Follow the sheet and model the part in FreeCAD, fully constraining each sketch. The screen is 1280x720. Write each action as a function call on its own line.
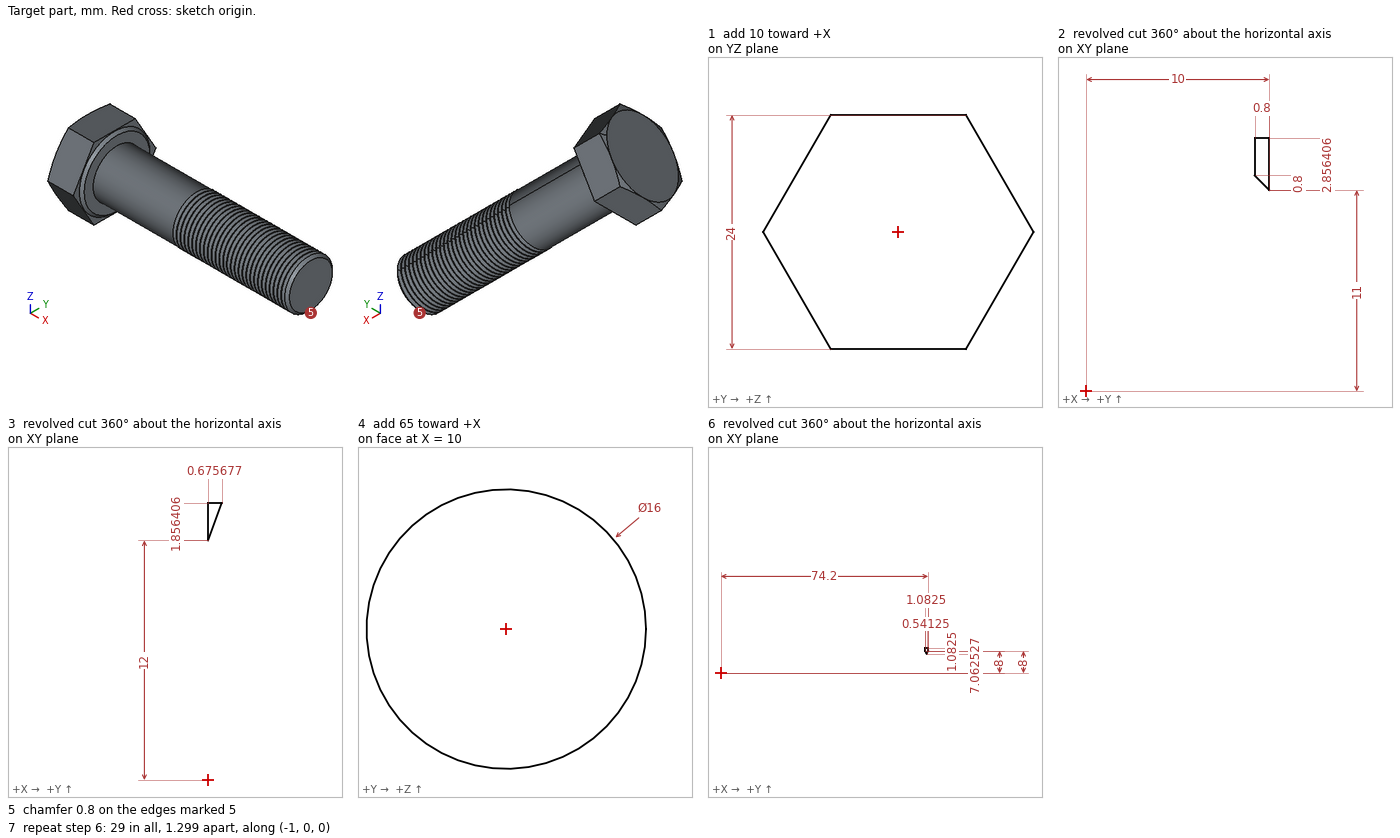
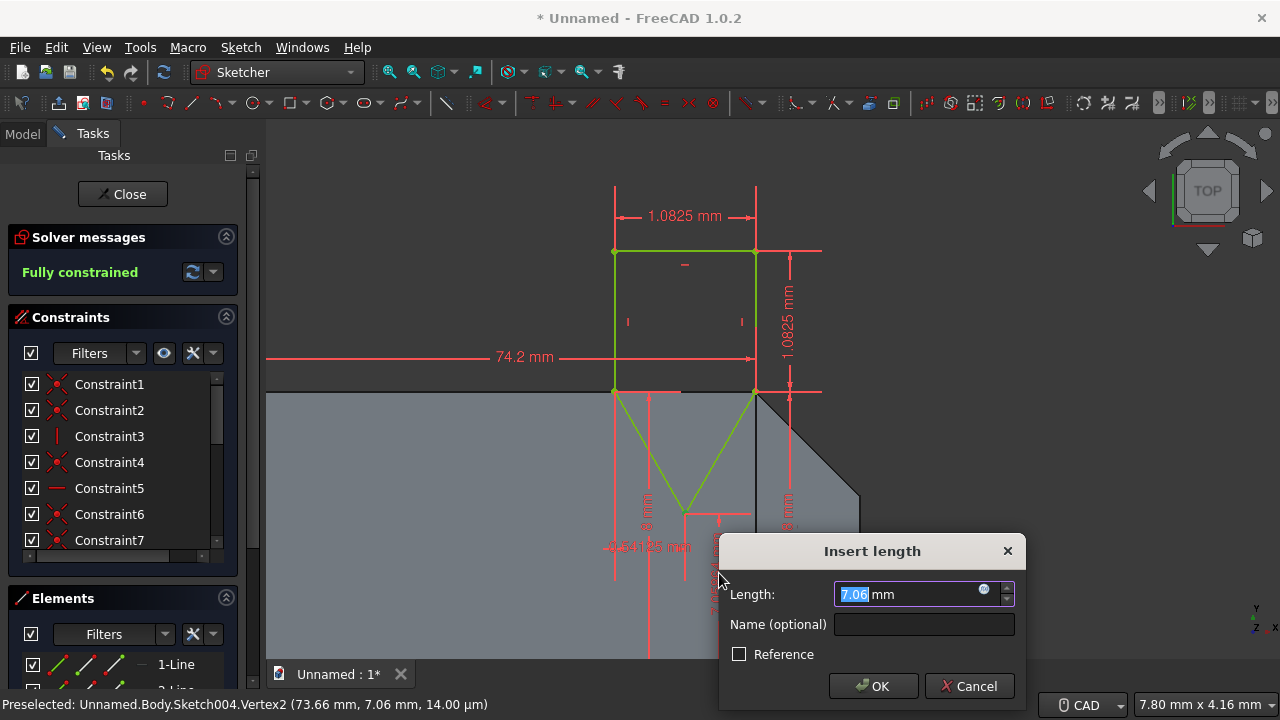
text(7.062527)
key(Return)
key(Escape)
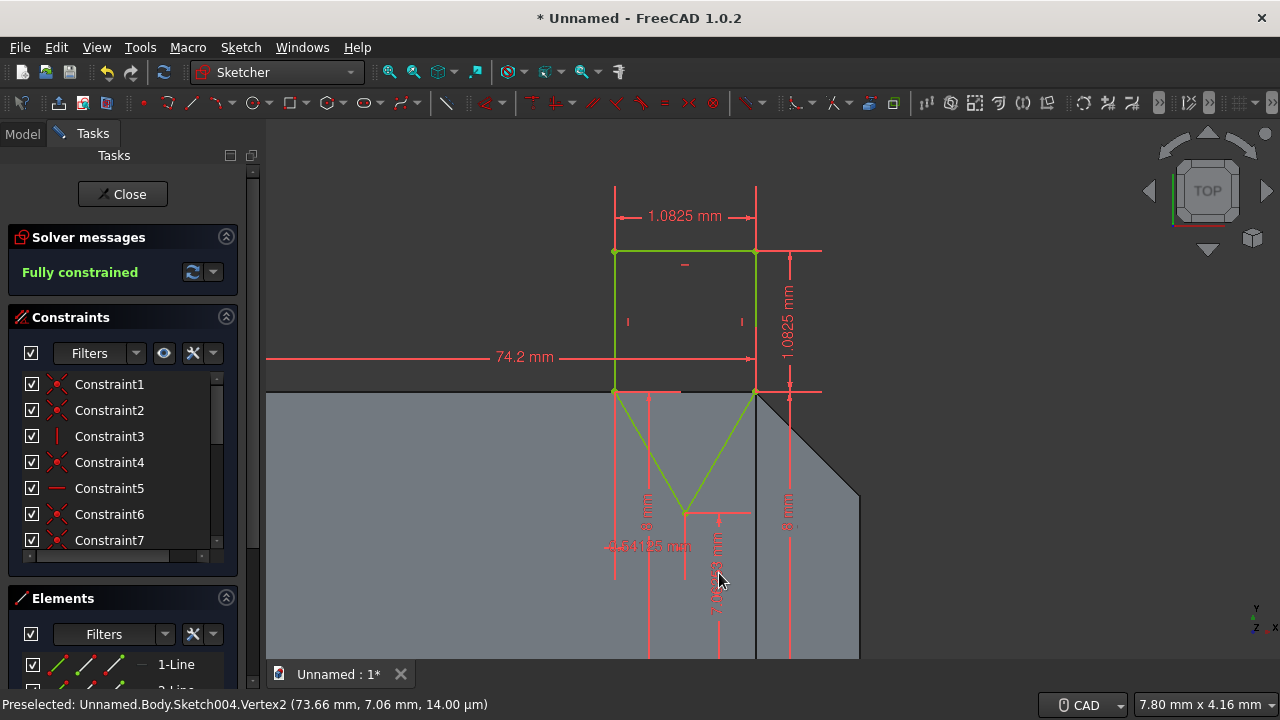
click(123, 194)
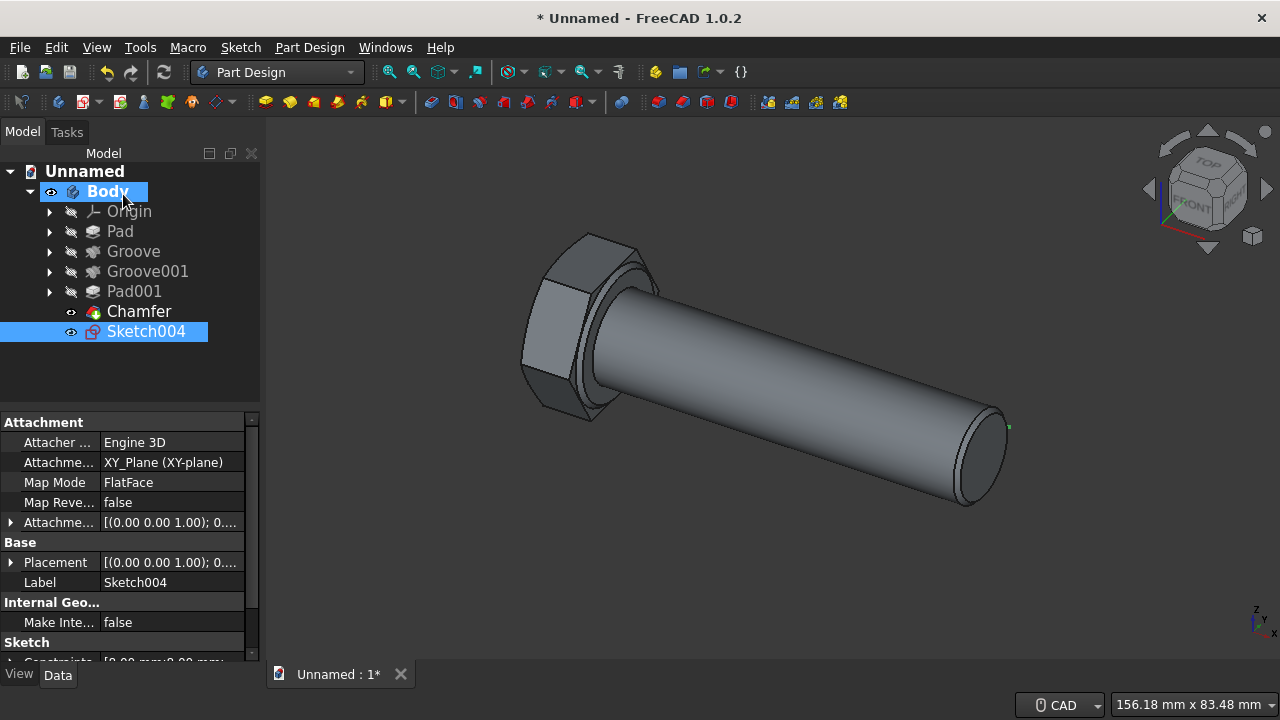
click(480, 102)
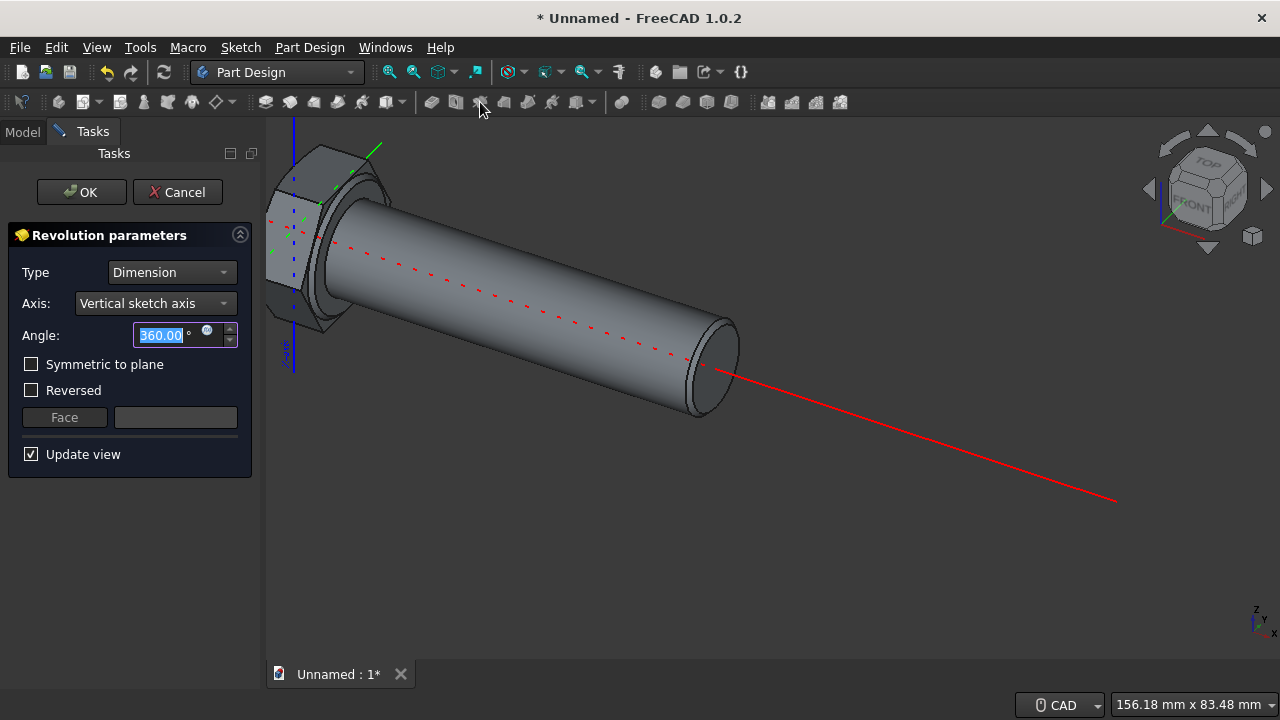
click(156, 304)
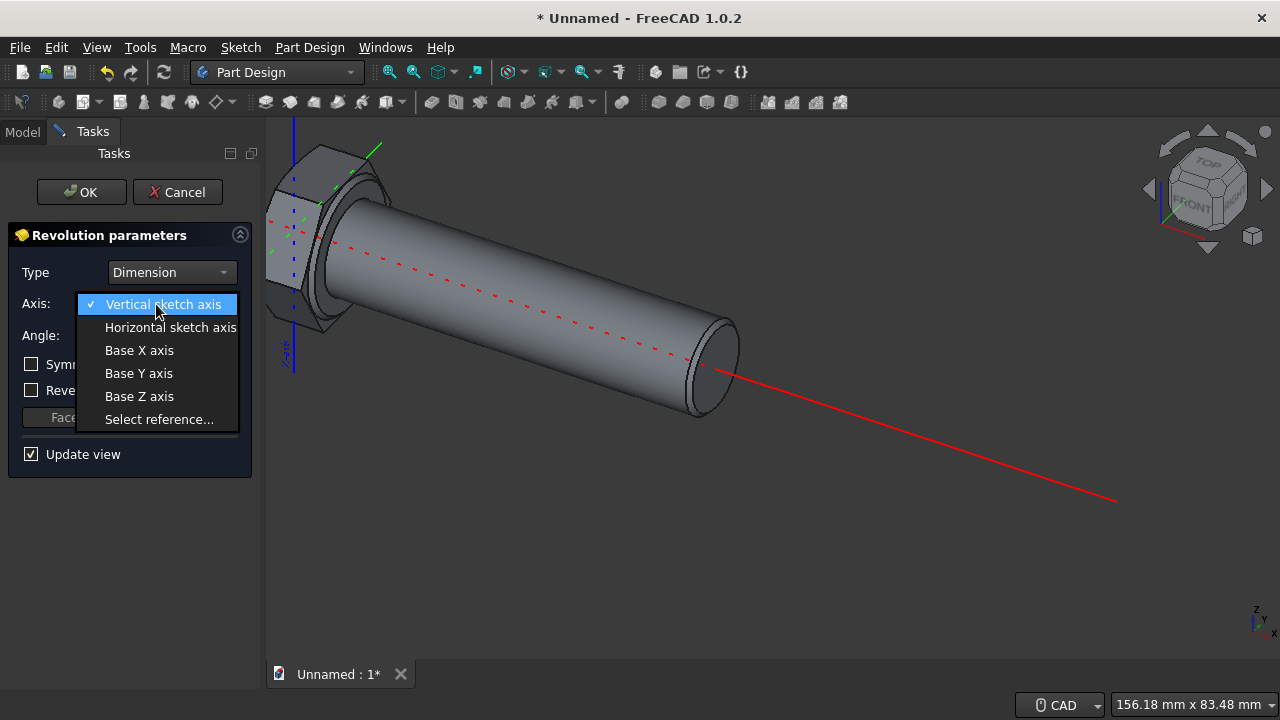
click(156, 328)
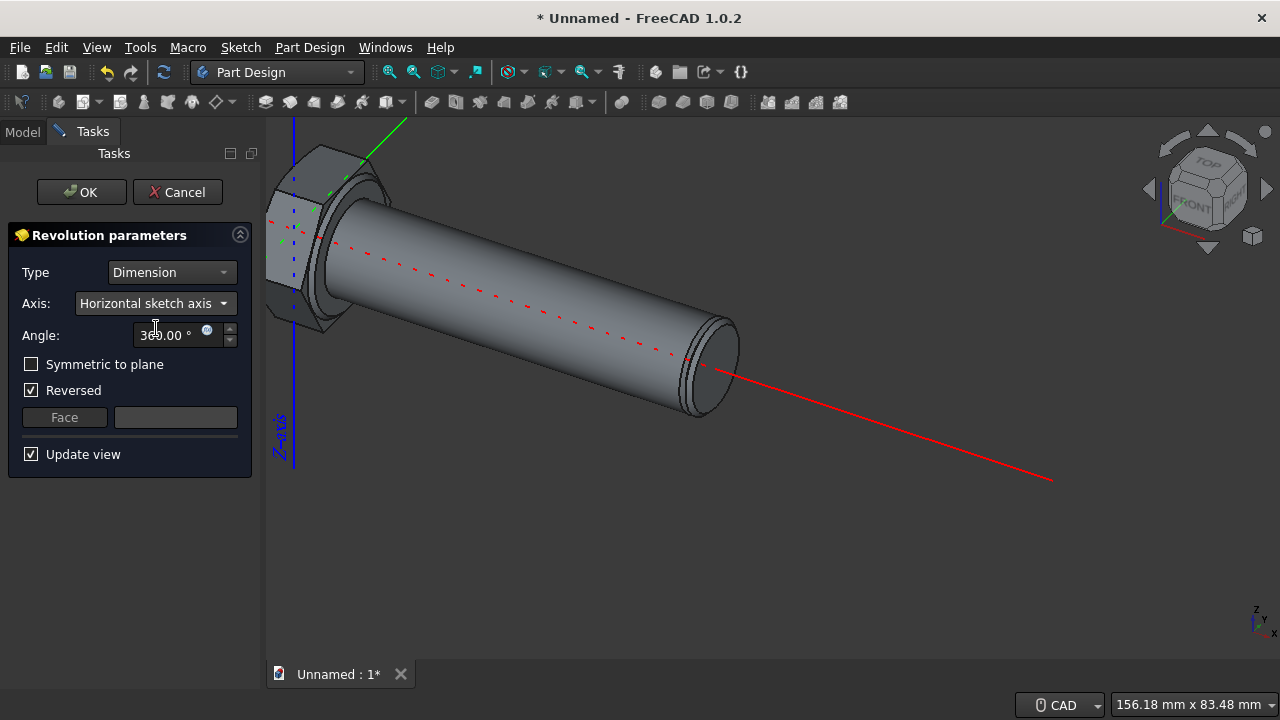
click(82, 192)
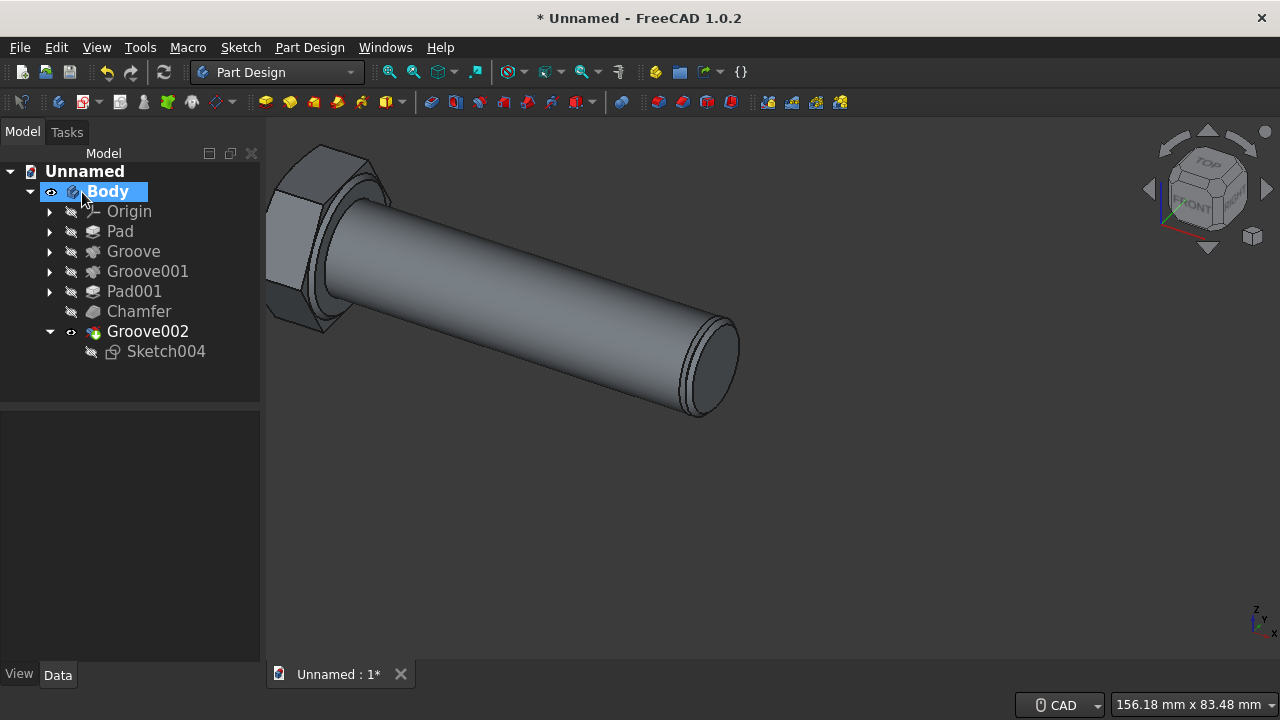
key(v)
key(f)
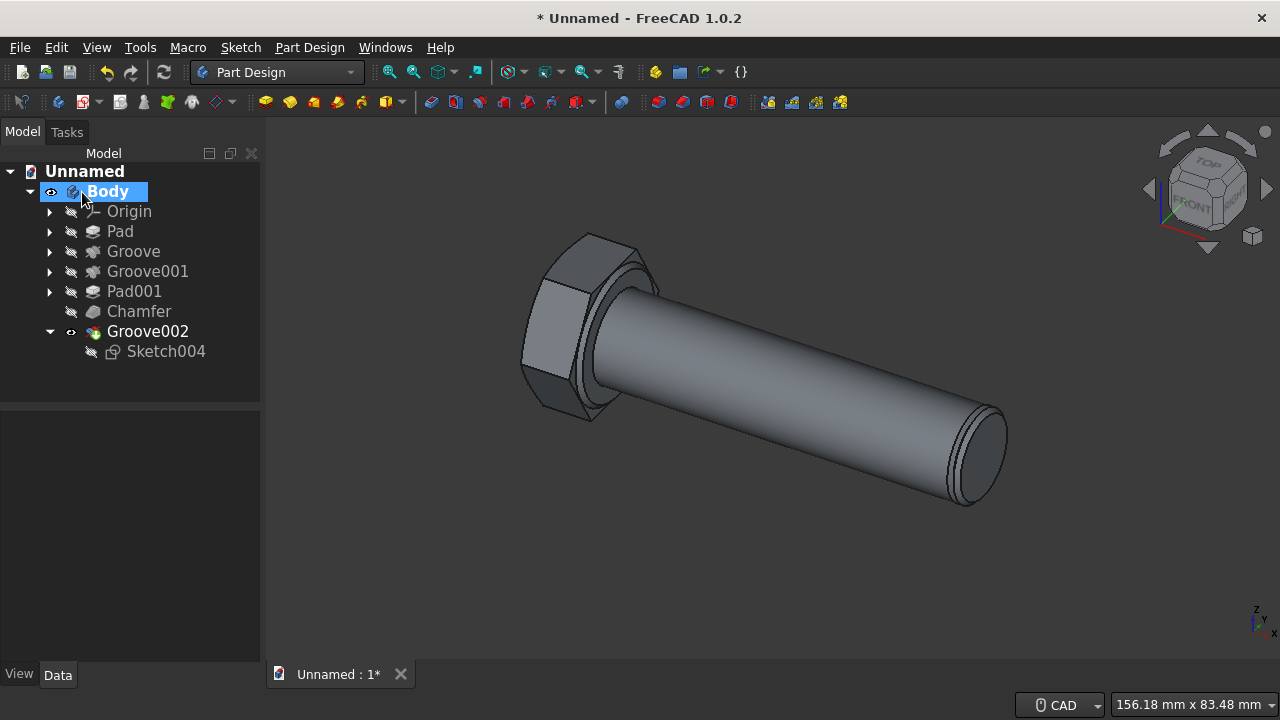
click(116, 332)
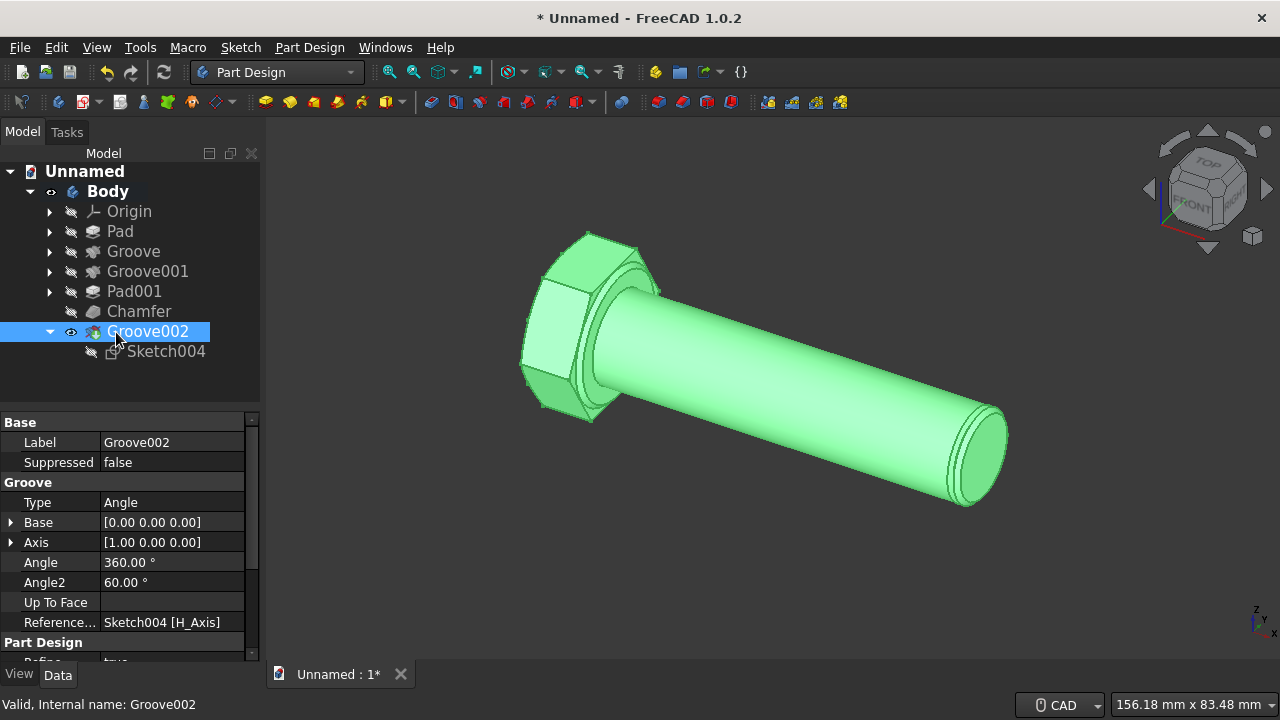
click(792, 102)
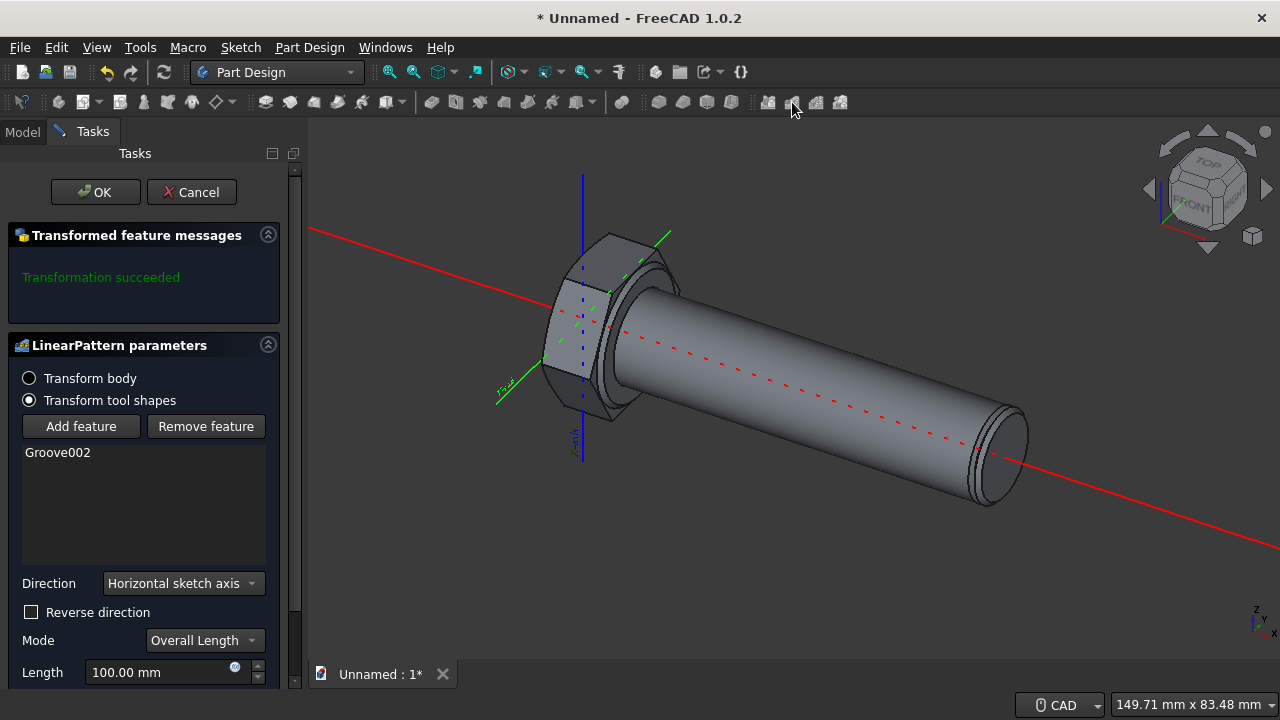
click(184, 584)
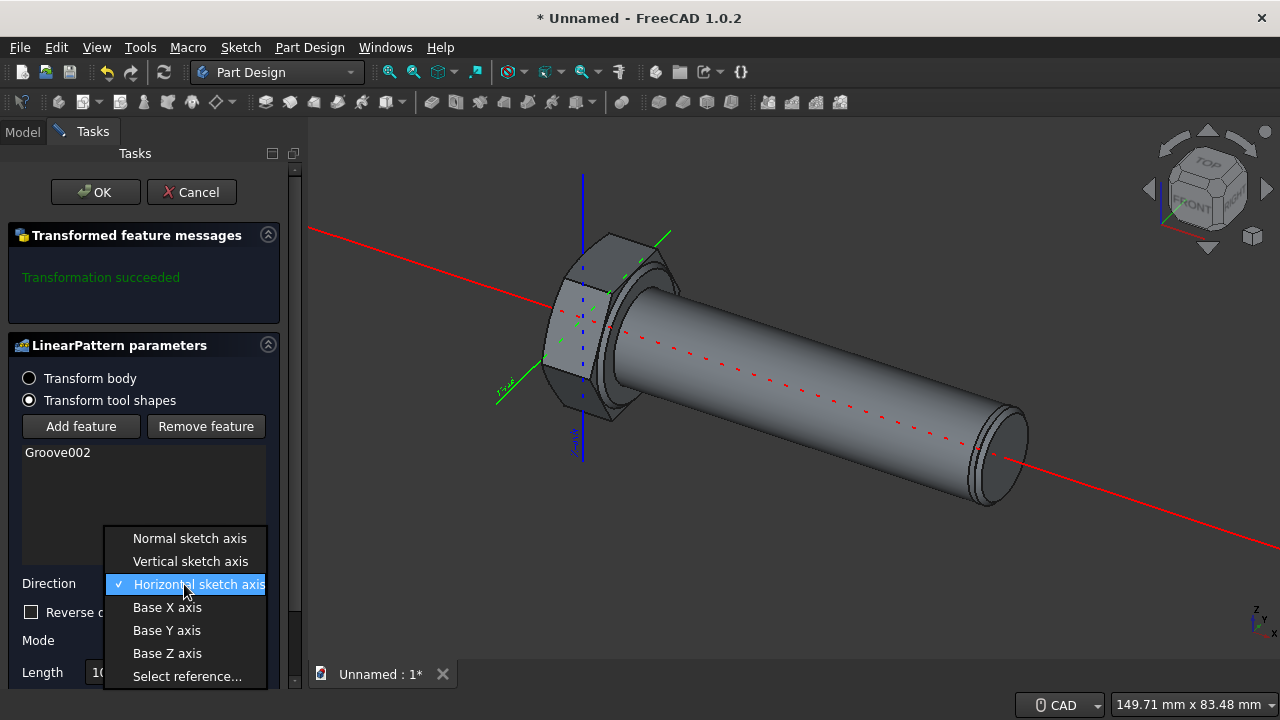
click(184, 608)